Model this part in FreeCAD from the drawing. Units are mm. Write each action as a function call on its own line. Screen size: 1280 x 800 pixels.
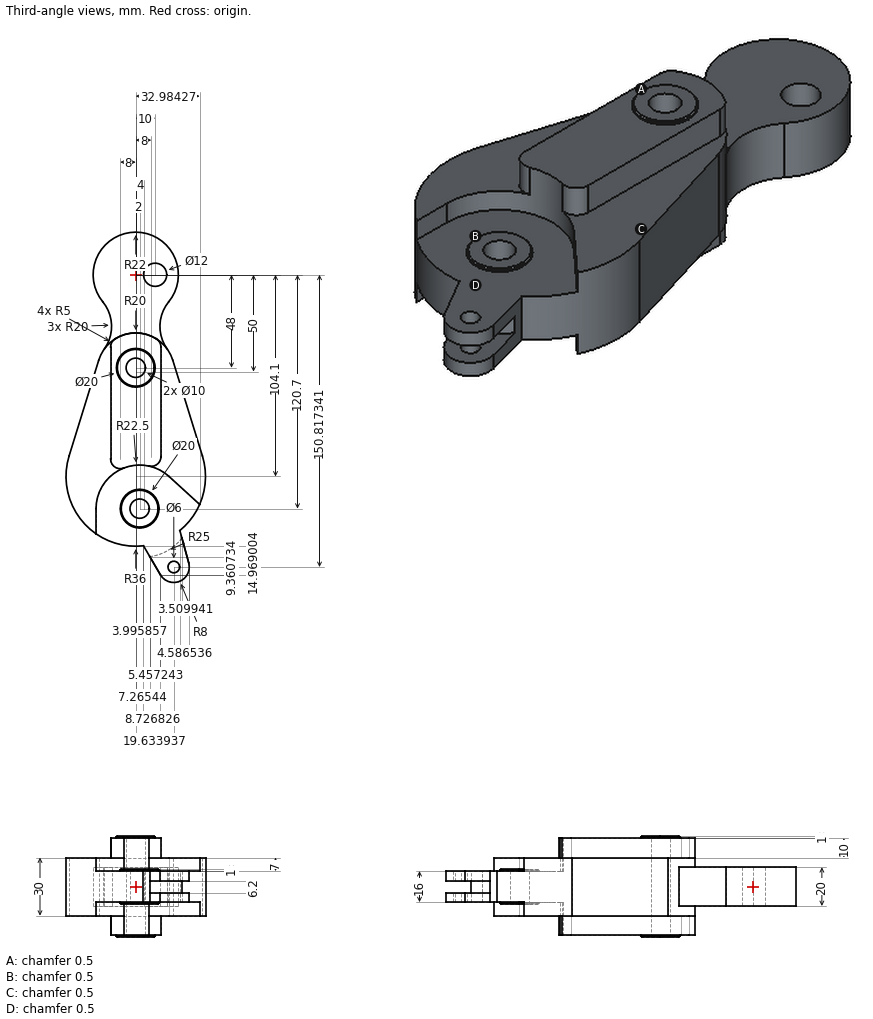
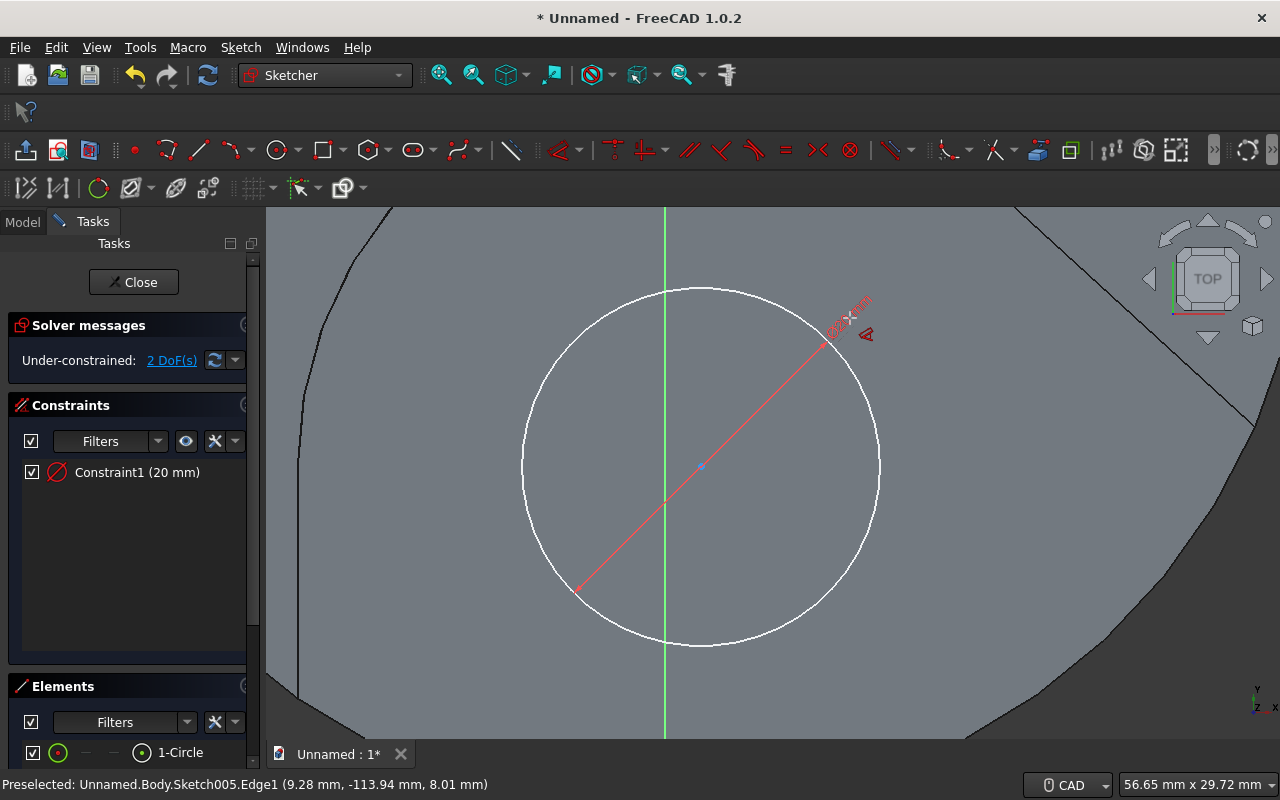
click(701, 467)
click(683, 501)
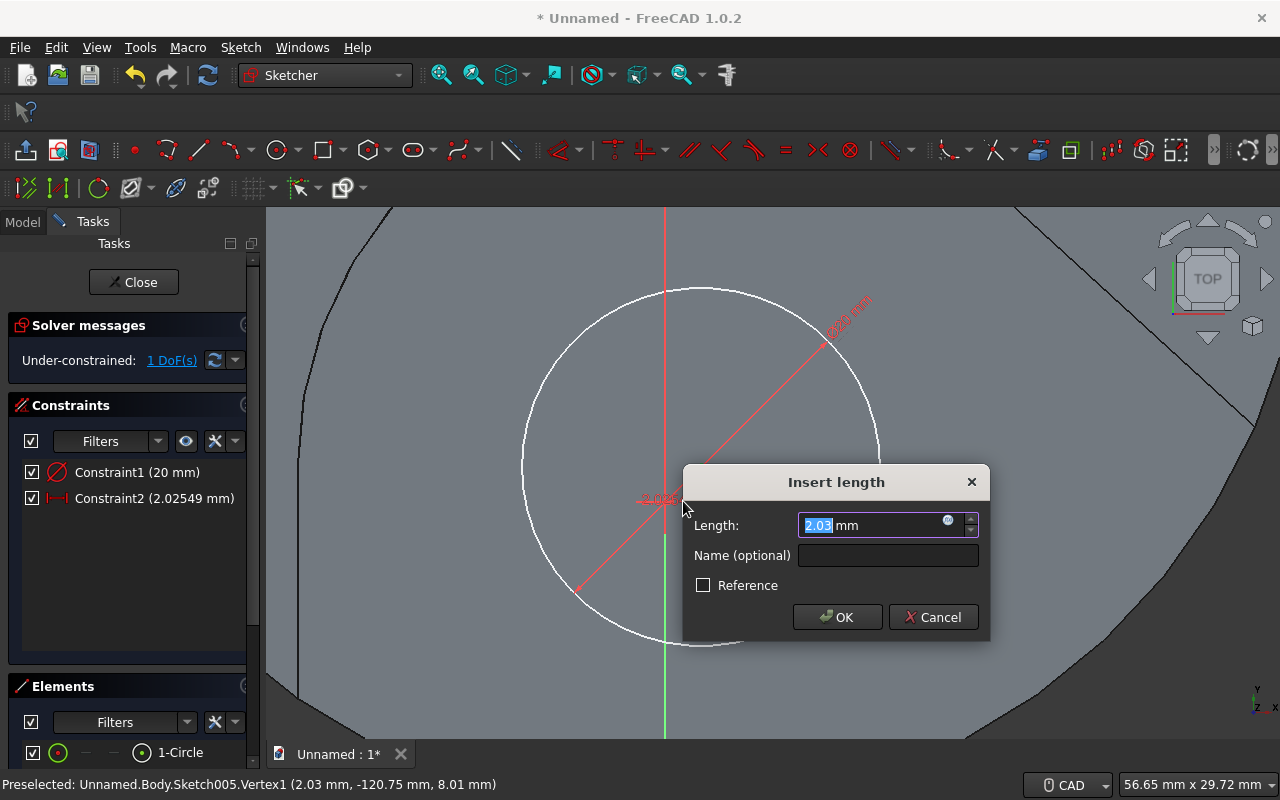
text(2)
key(Return)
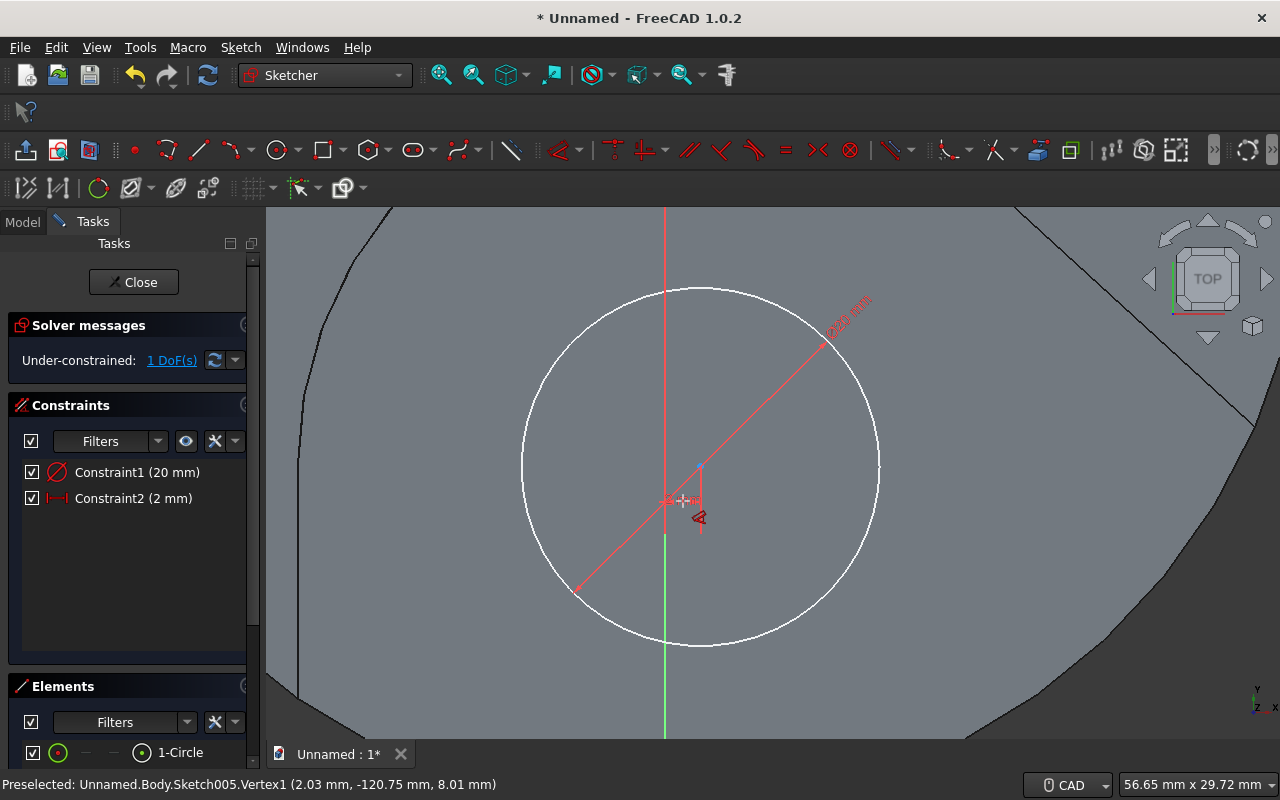
click(701, 467)
click(631, 351)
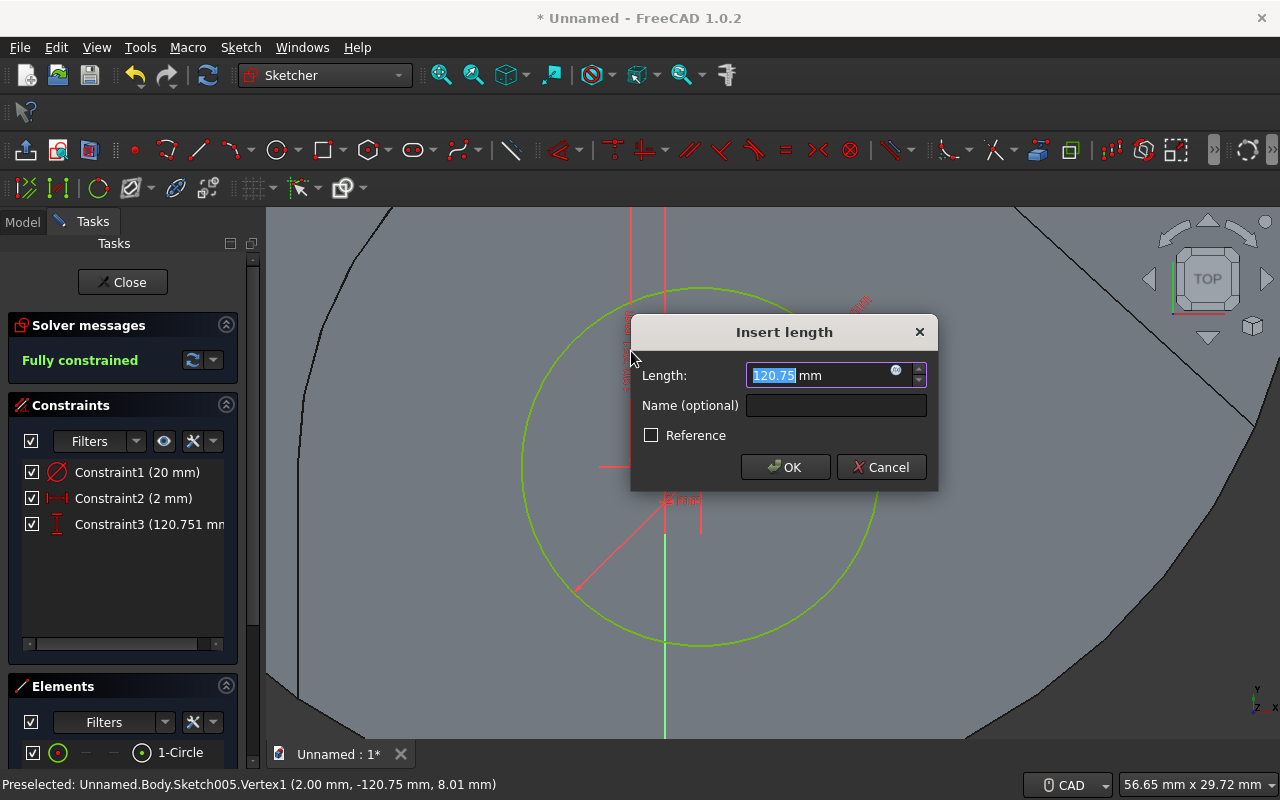
text(120.7)
key(Return)
key(Escape)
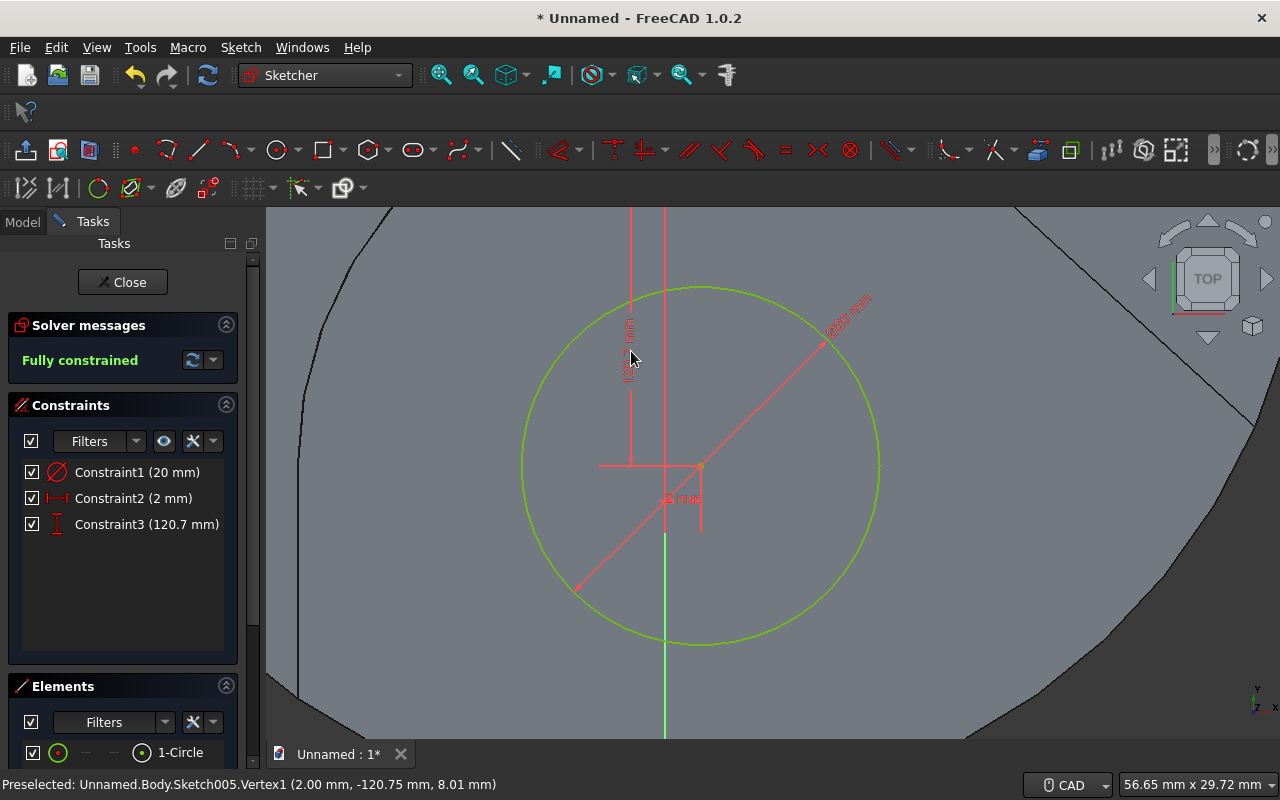
click(123, 282)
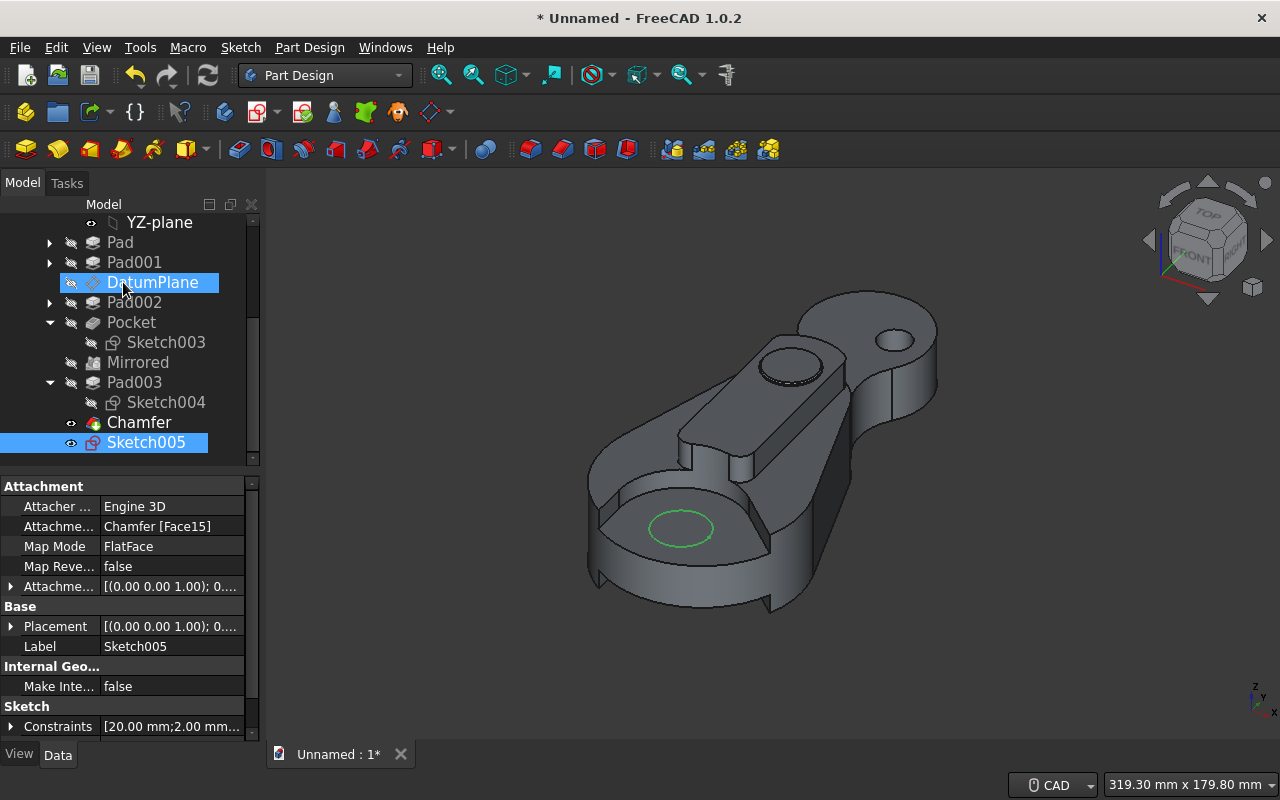
click(26, 150)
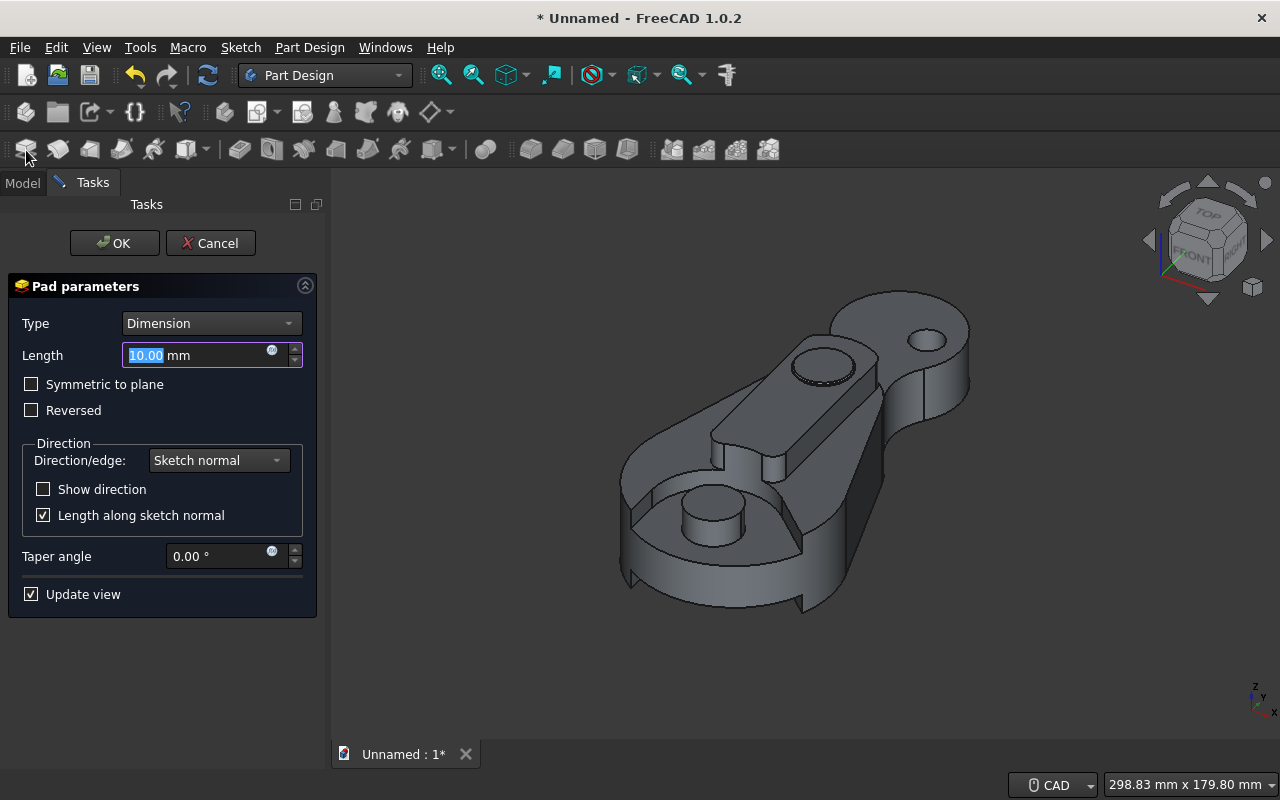
text(1)
key(Tab)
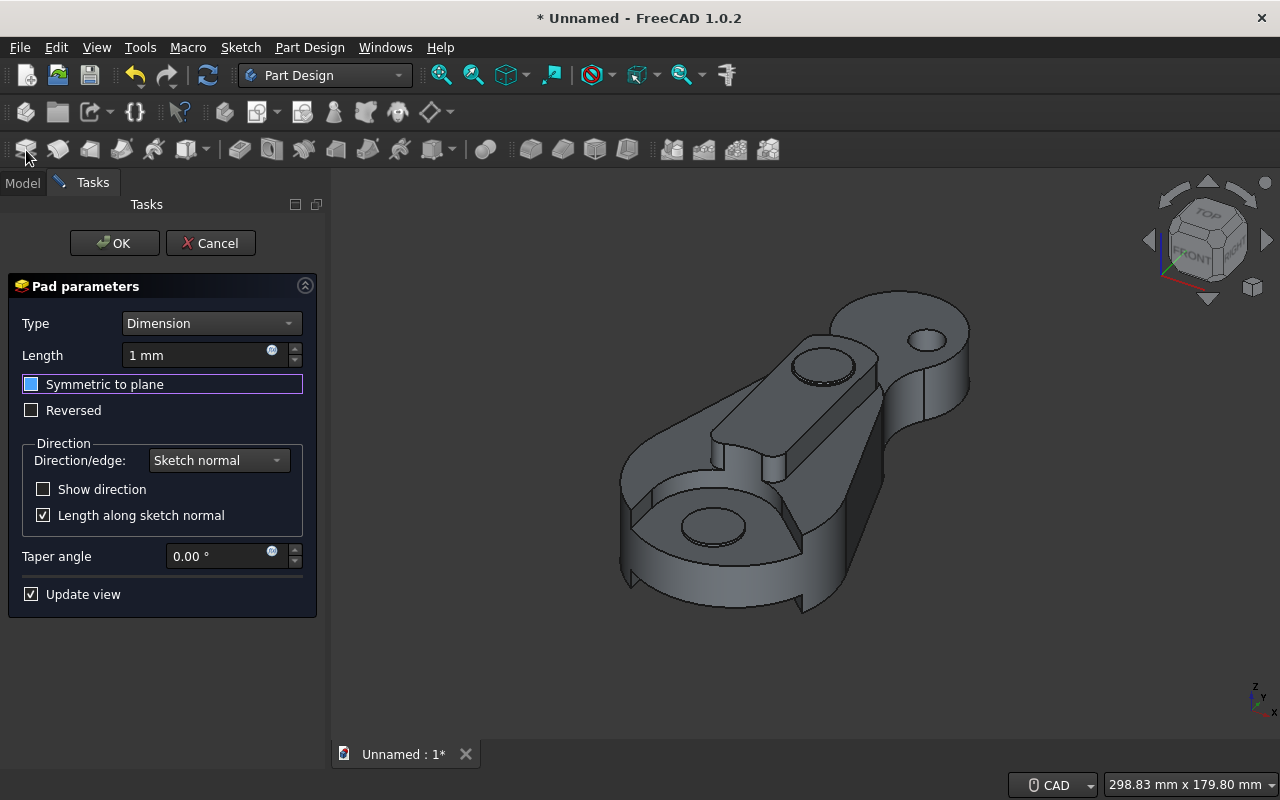
click(115, 243)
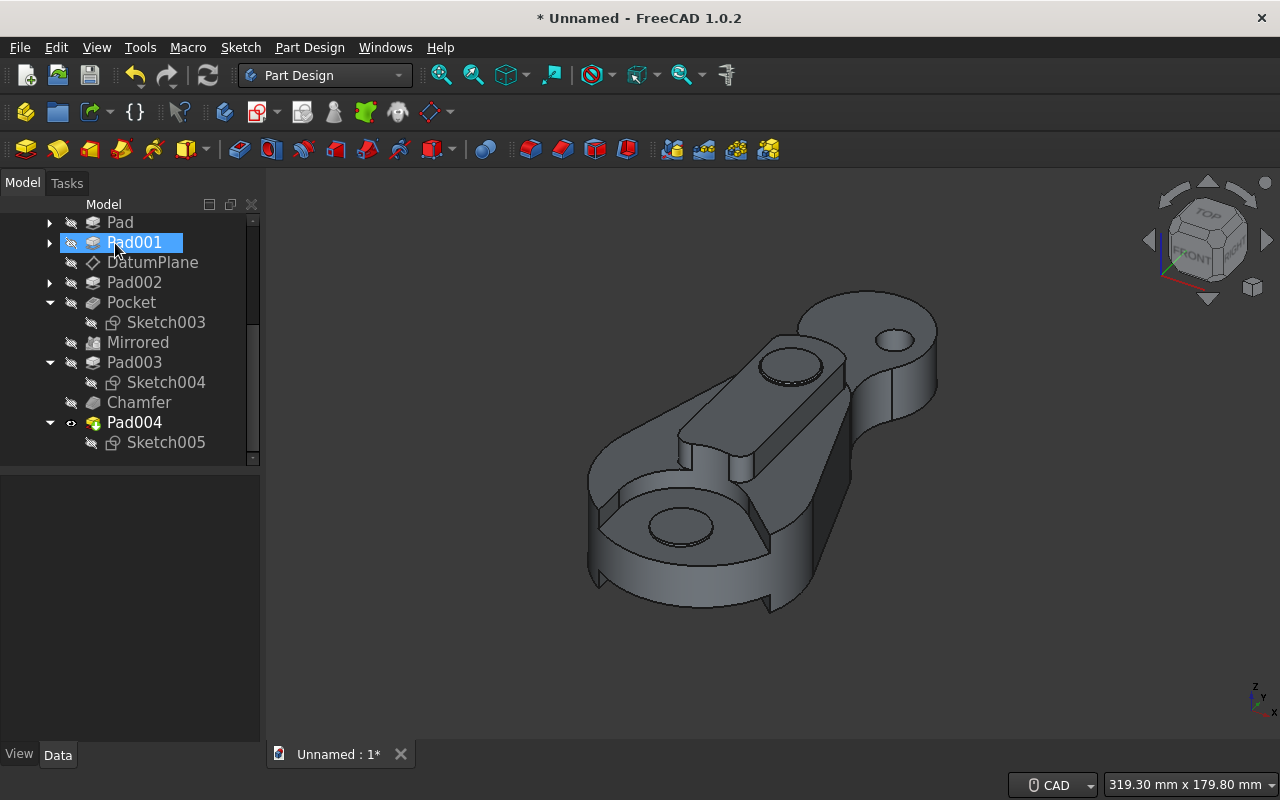
click(649, 527)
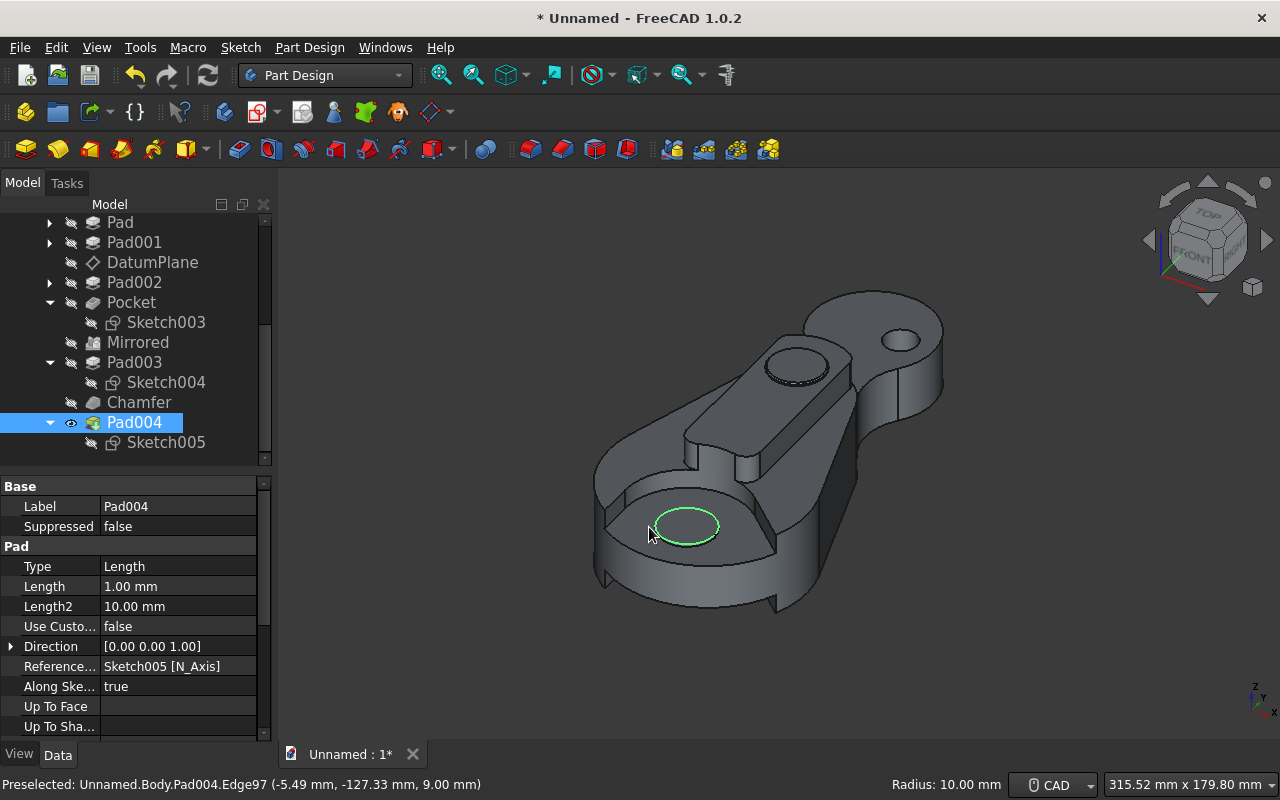
click(564, 150)